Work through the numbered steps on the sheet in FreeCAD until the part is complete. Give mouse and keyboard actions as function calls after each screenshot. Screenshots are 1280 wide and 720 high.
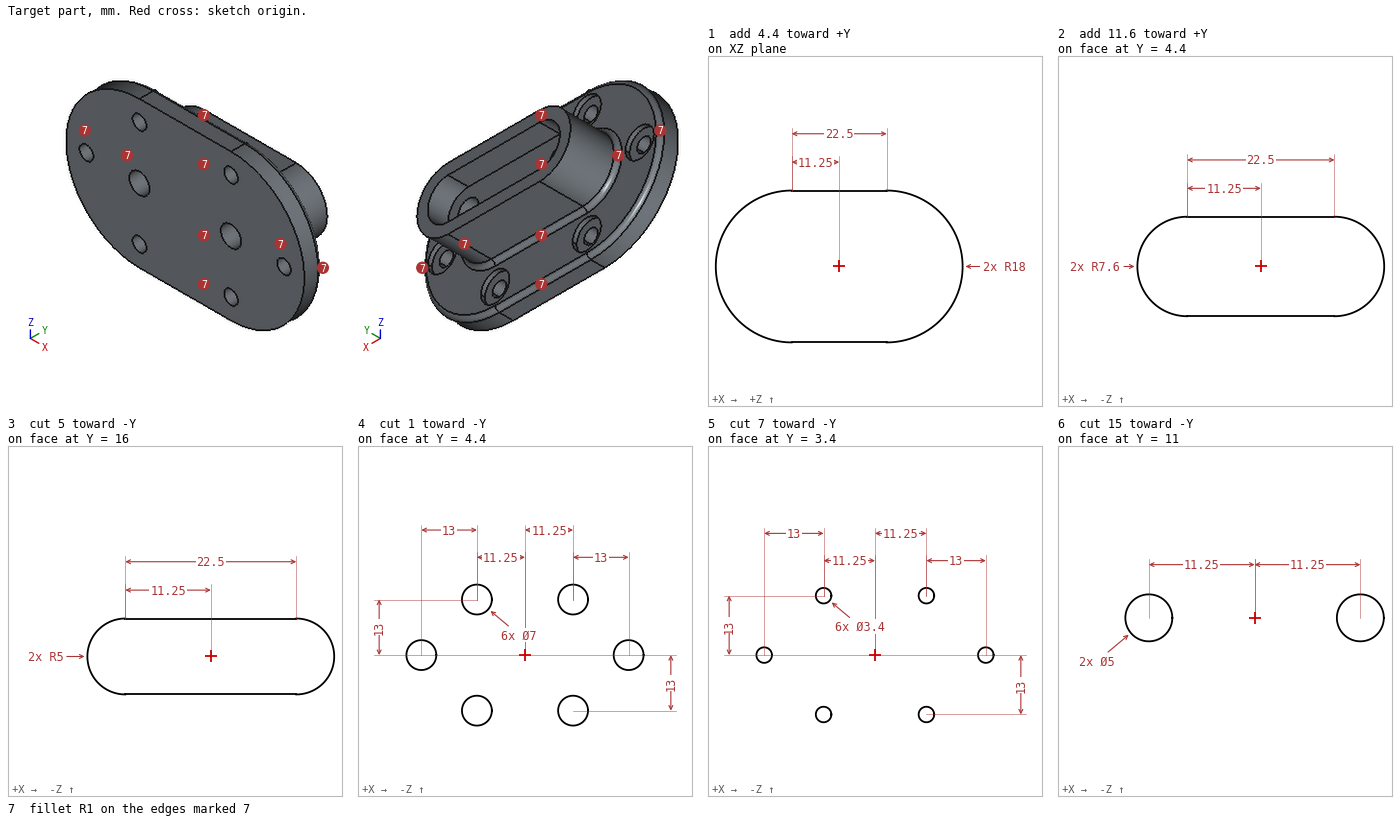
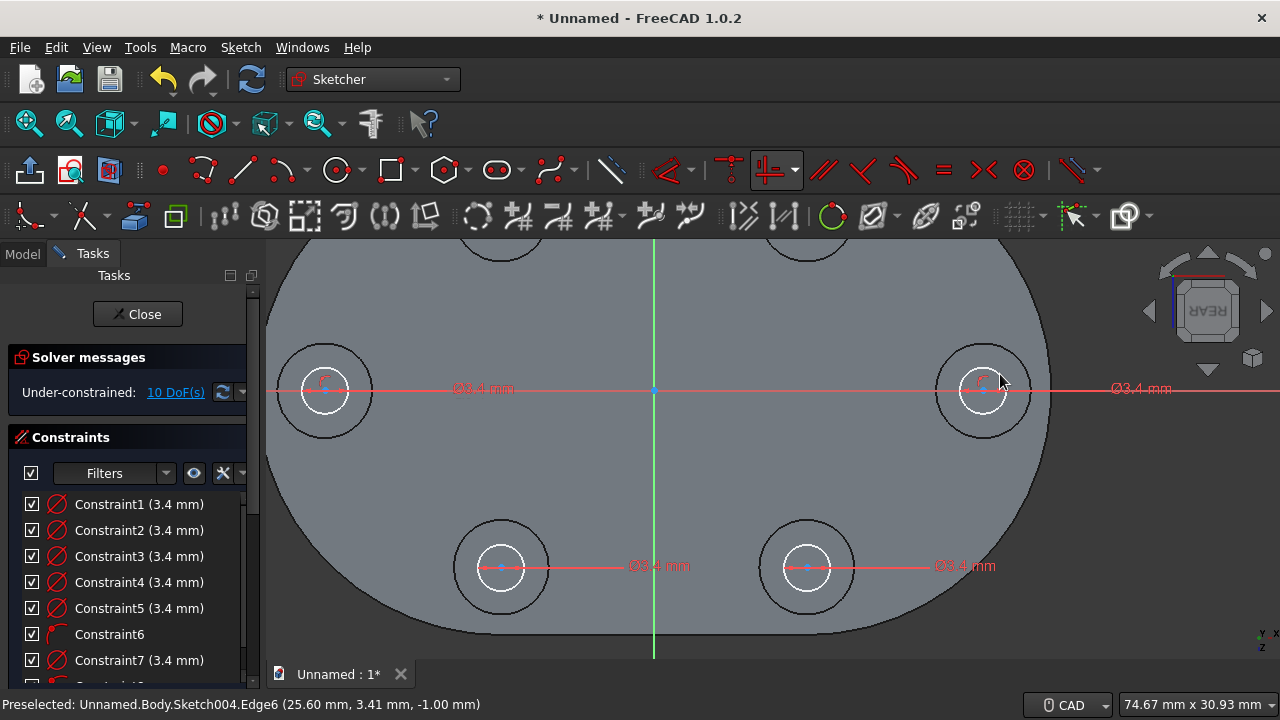
scroll(807, 568, down, 2)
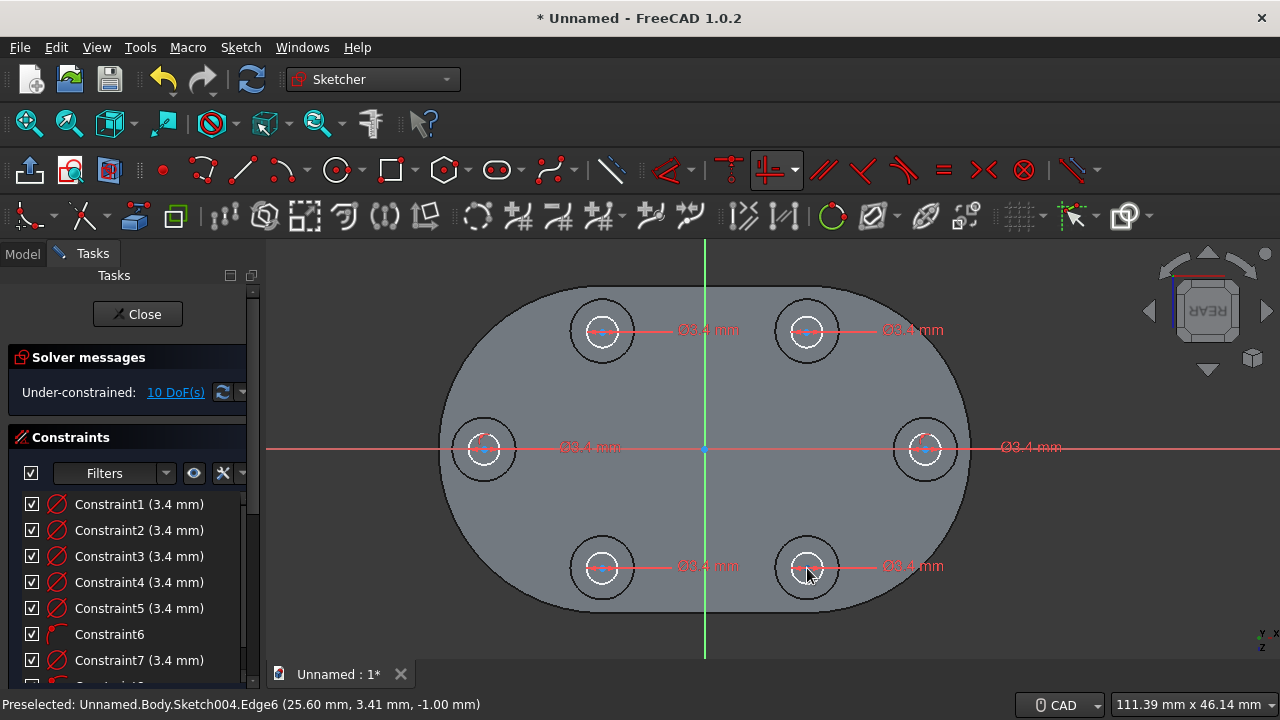
click(602, 332)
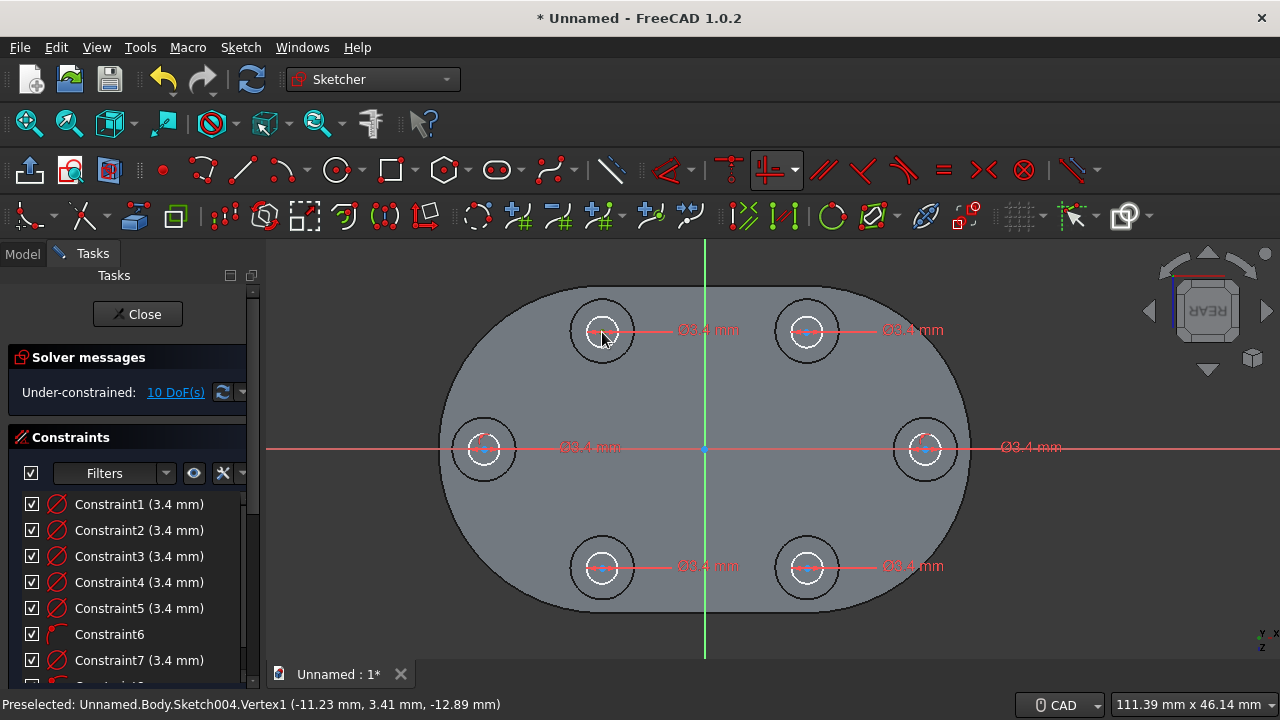
click(807, 332)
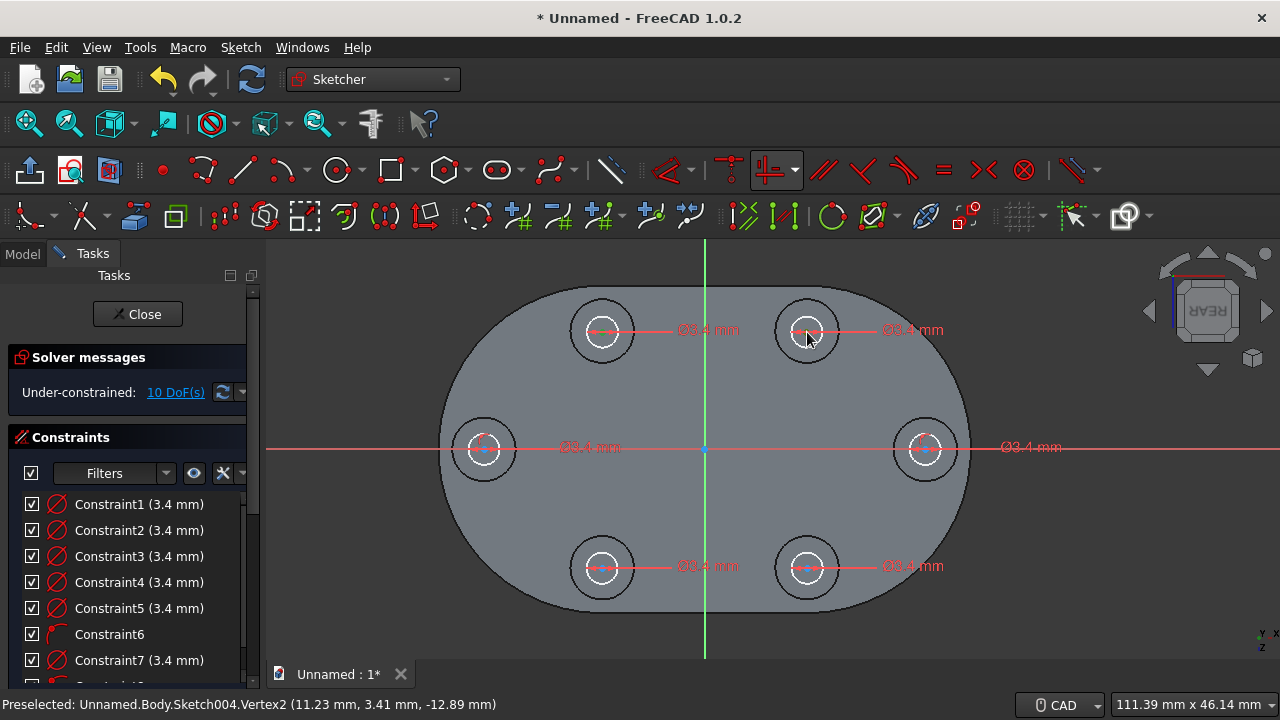
click(798, 170)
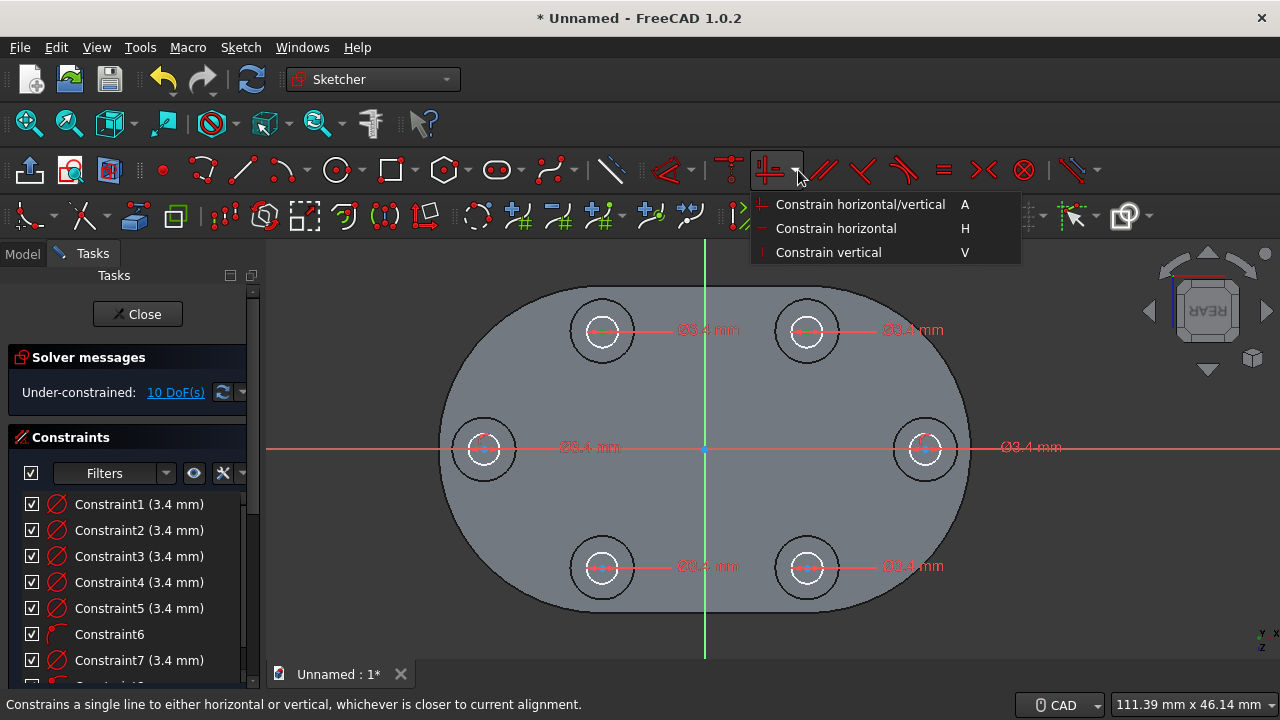
click(886, 228)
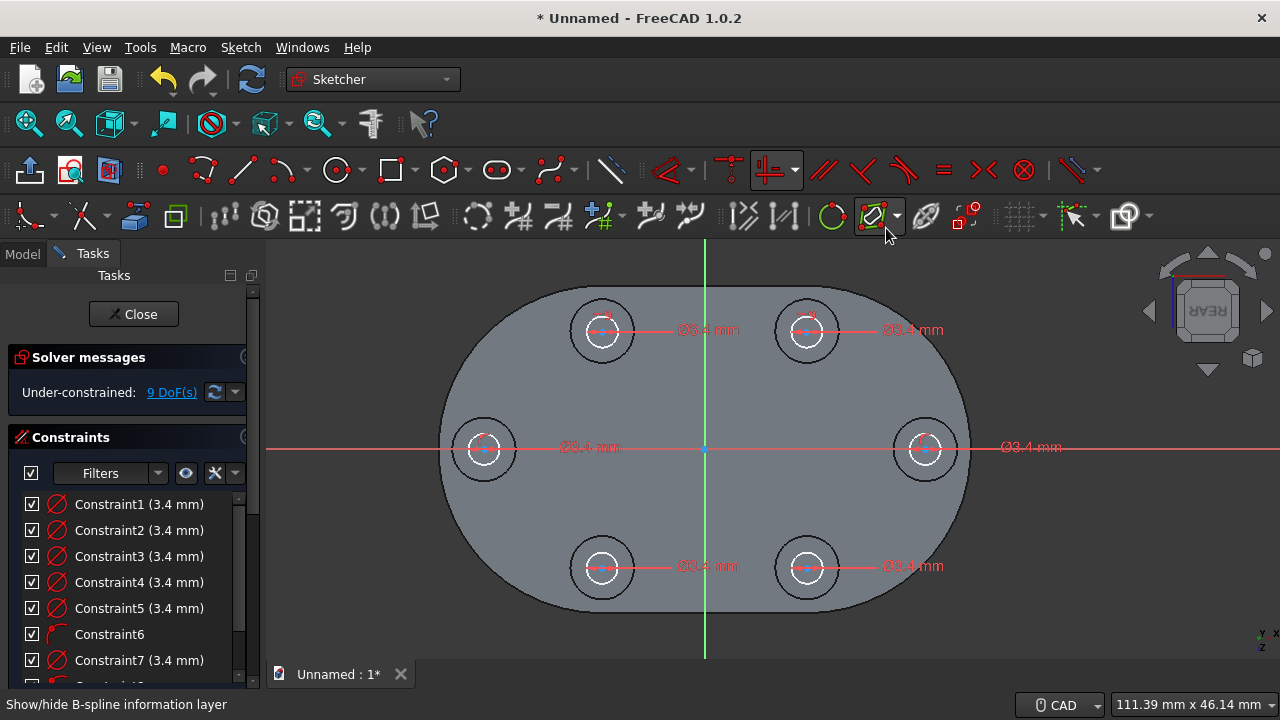
click(807, 332)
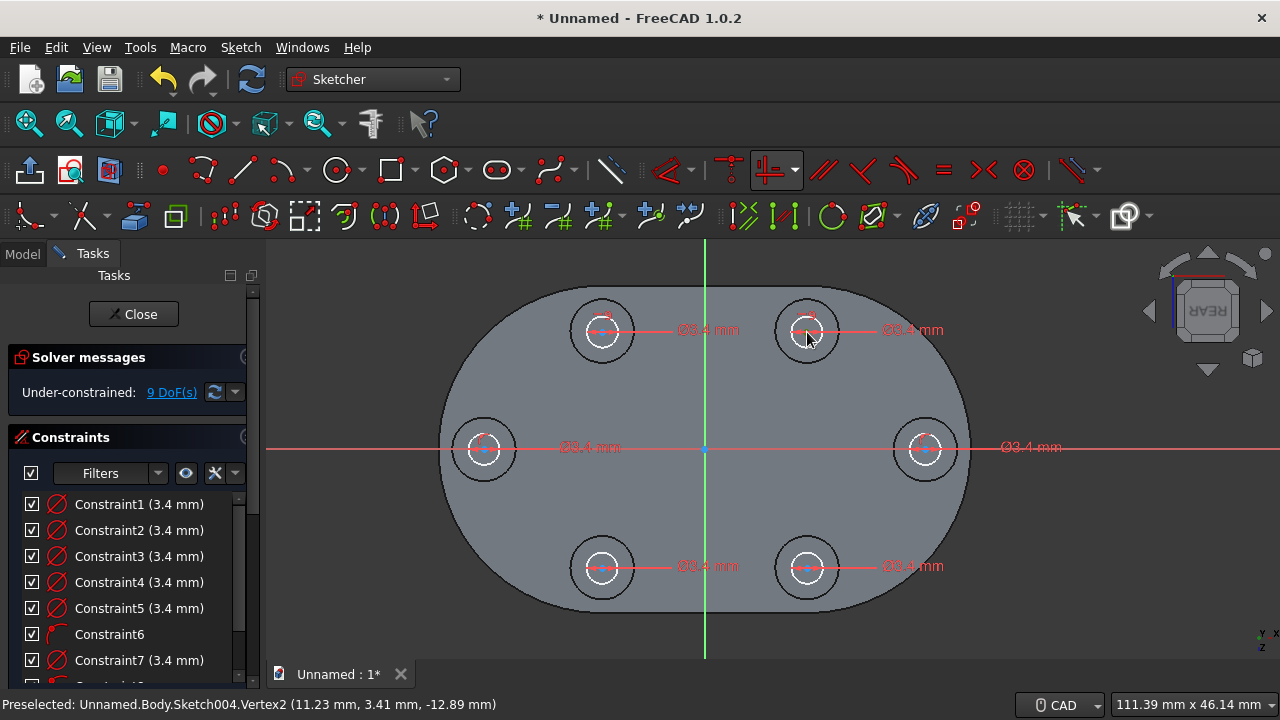
click(807, 568)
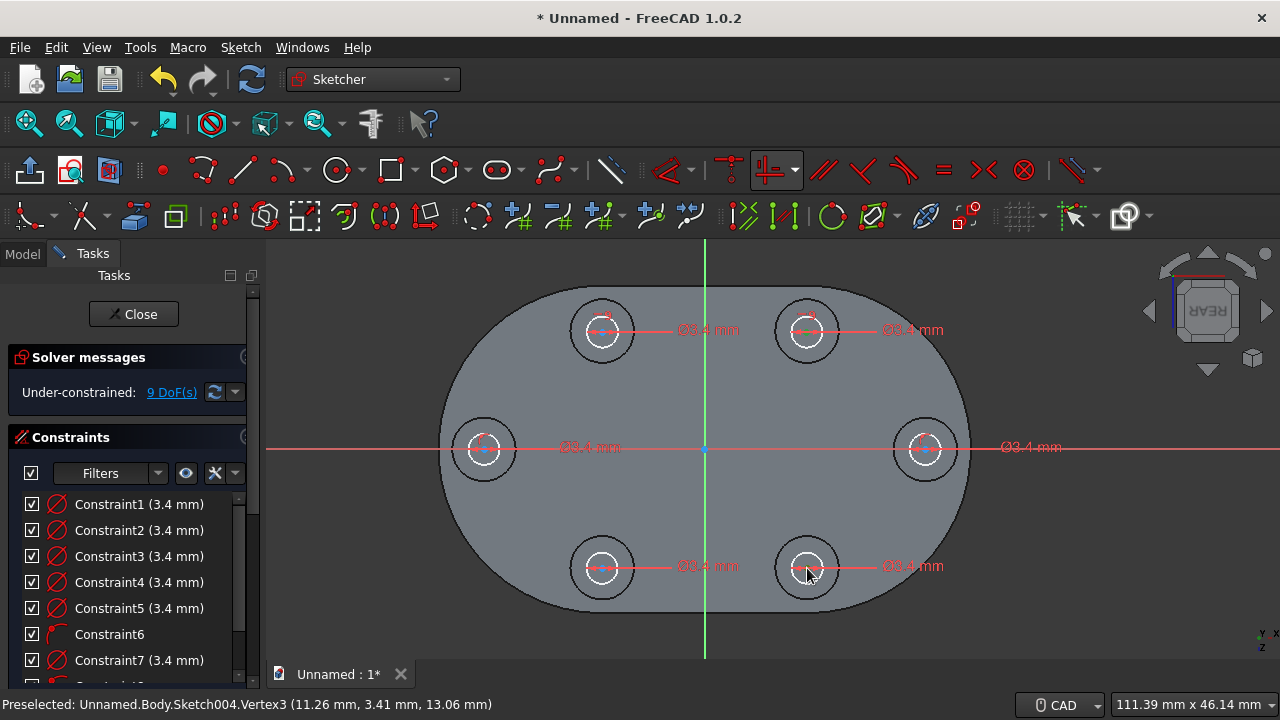
click(798, 170)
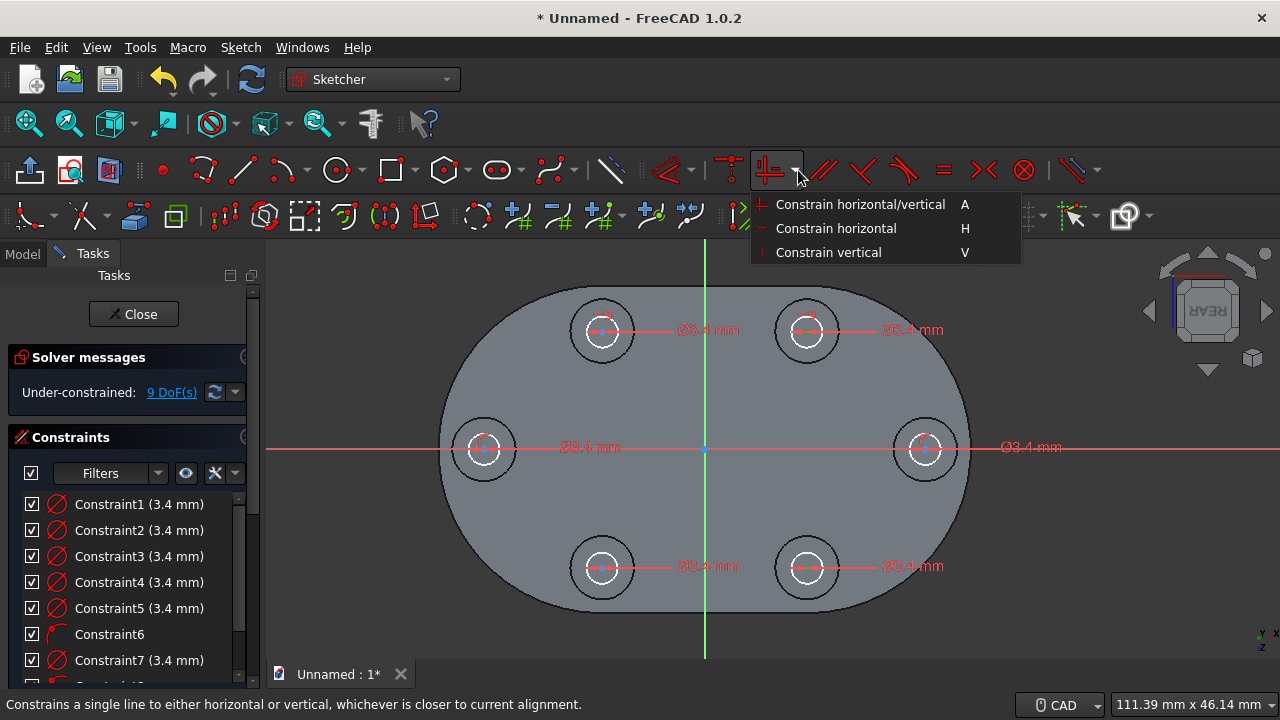
click(886, 252)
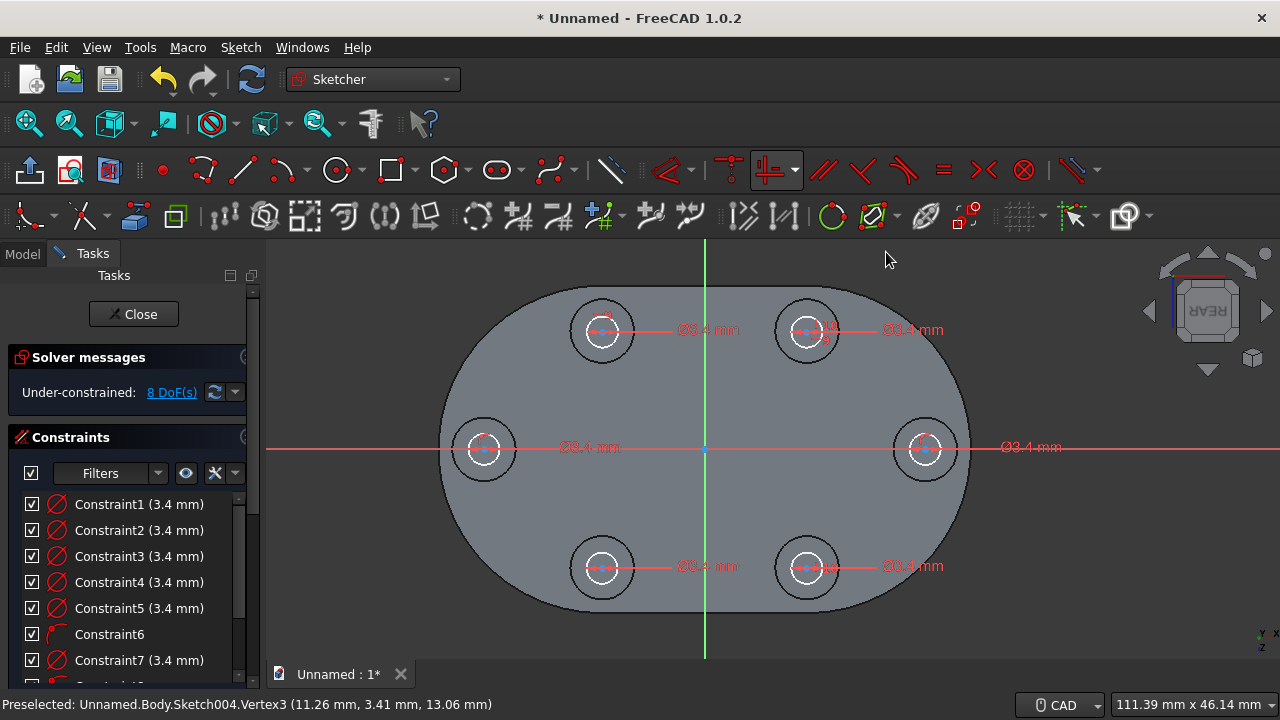
click(602, 332)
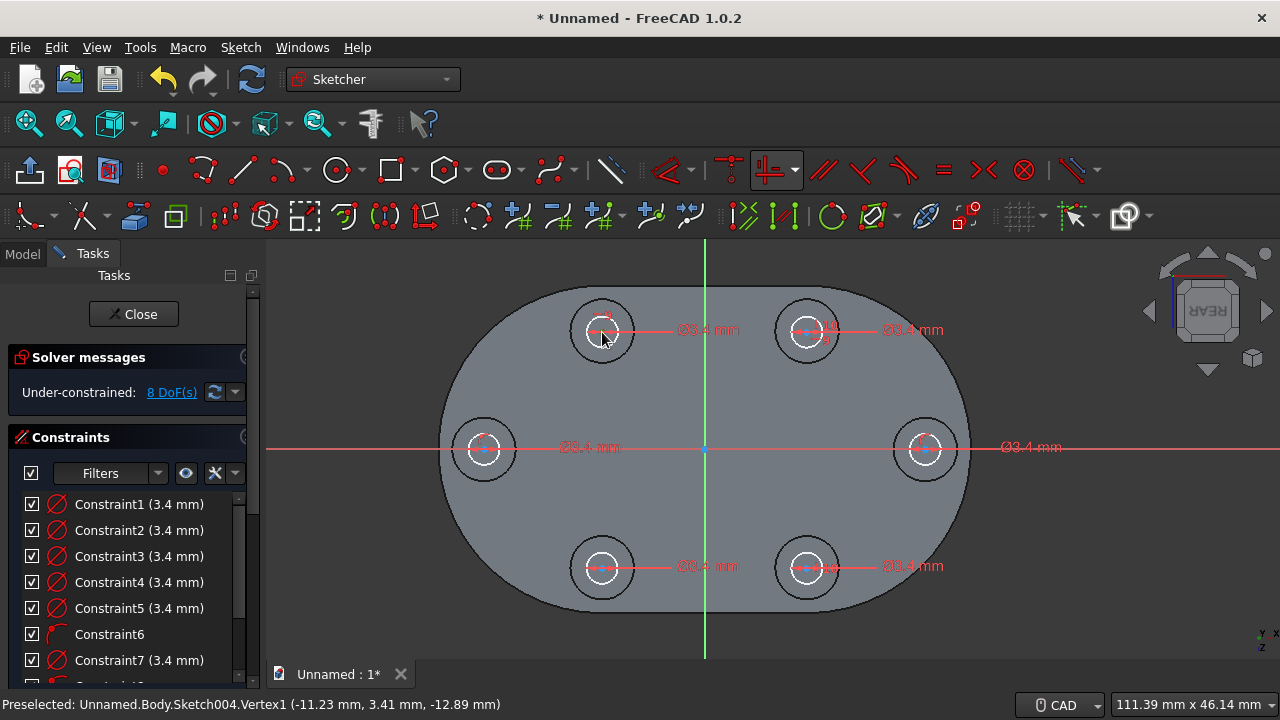
click(602, 568)